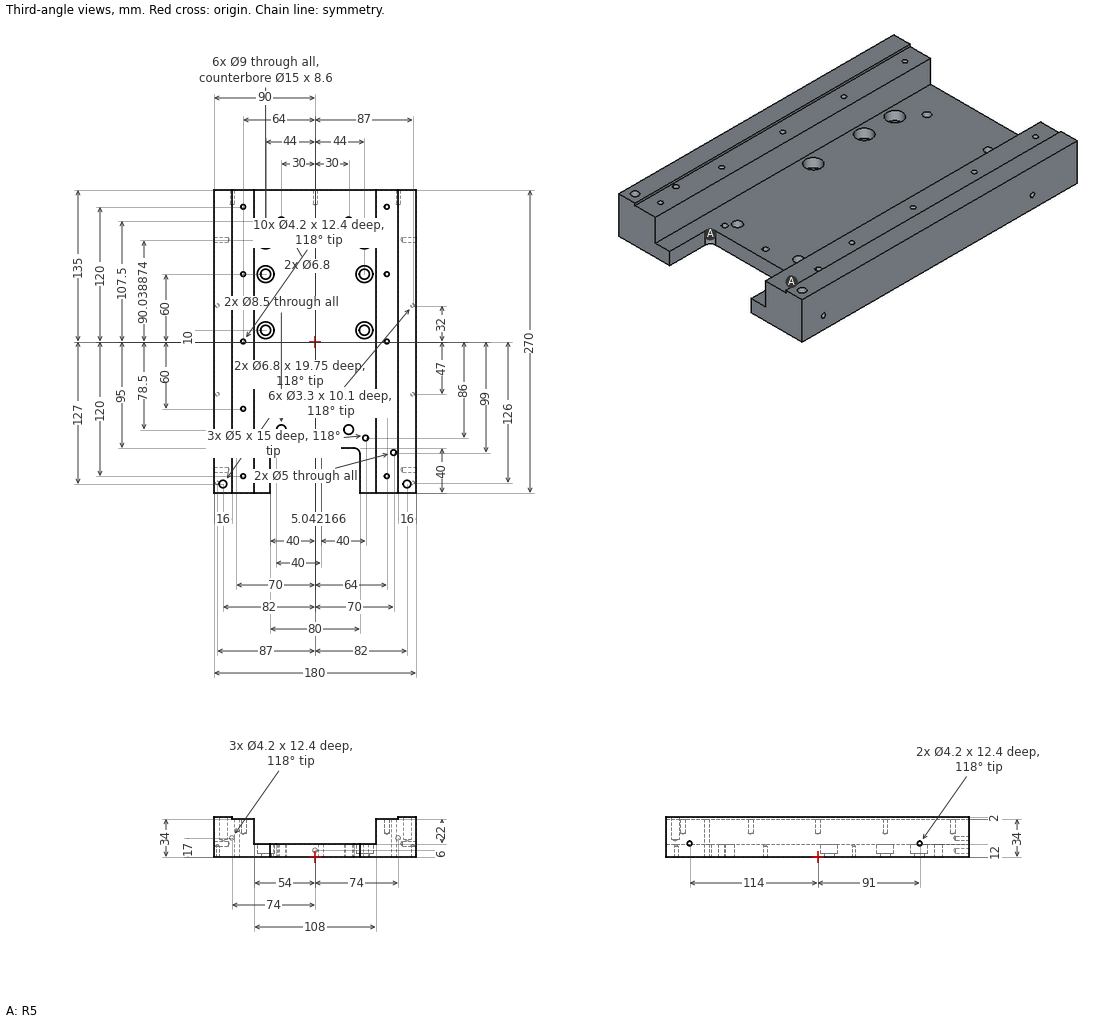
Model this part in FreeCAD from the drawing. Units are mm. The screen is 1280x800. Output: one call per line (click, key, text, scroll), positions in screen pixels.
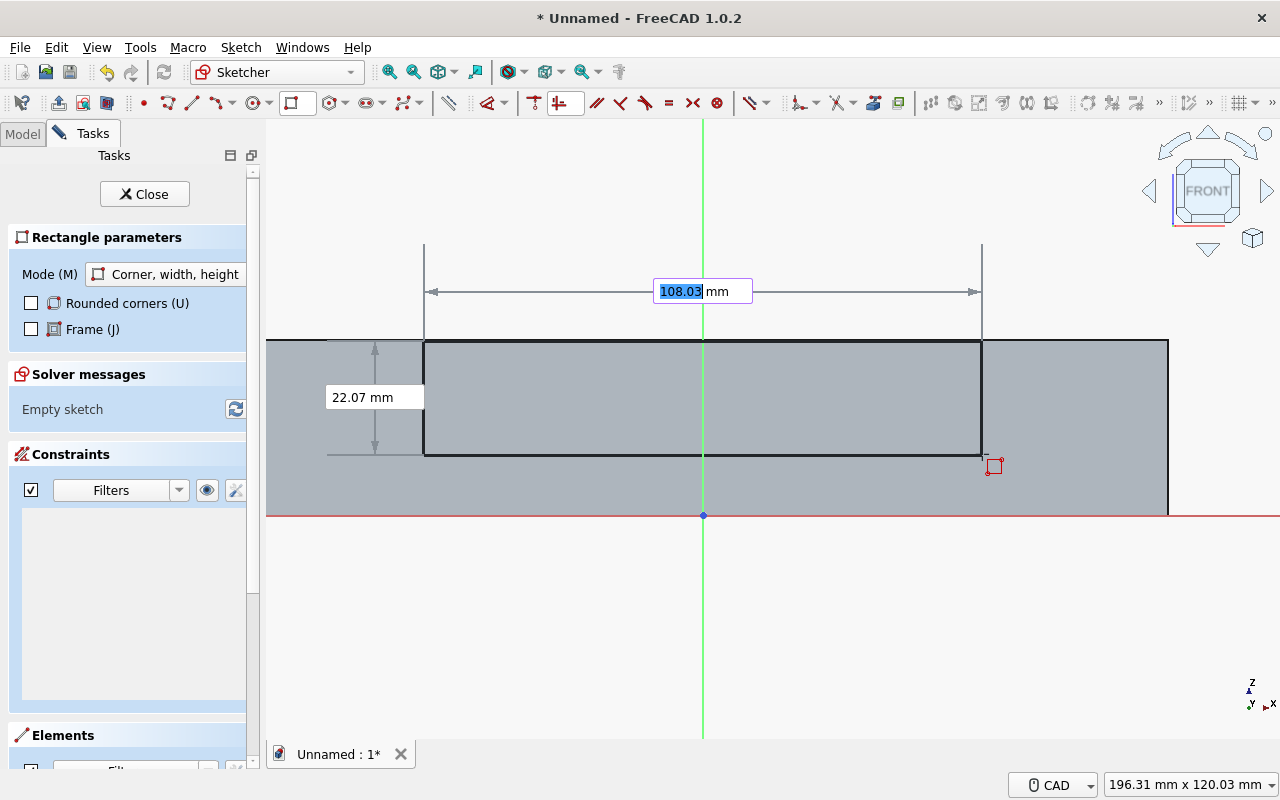
text(108)
key(Tab)
text(22)
key(Return)
key(Escape)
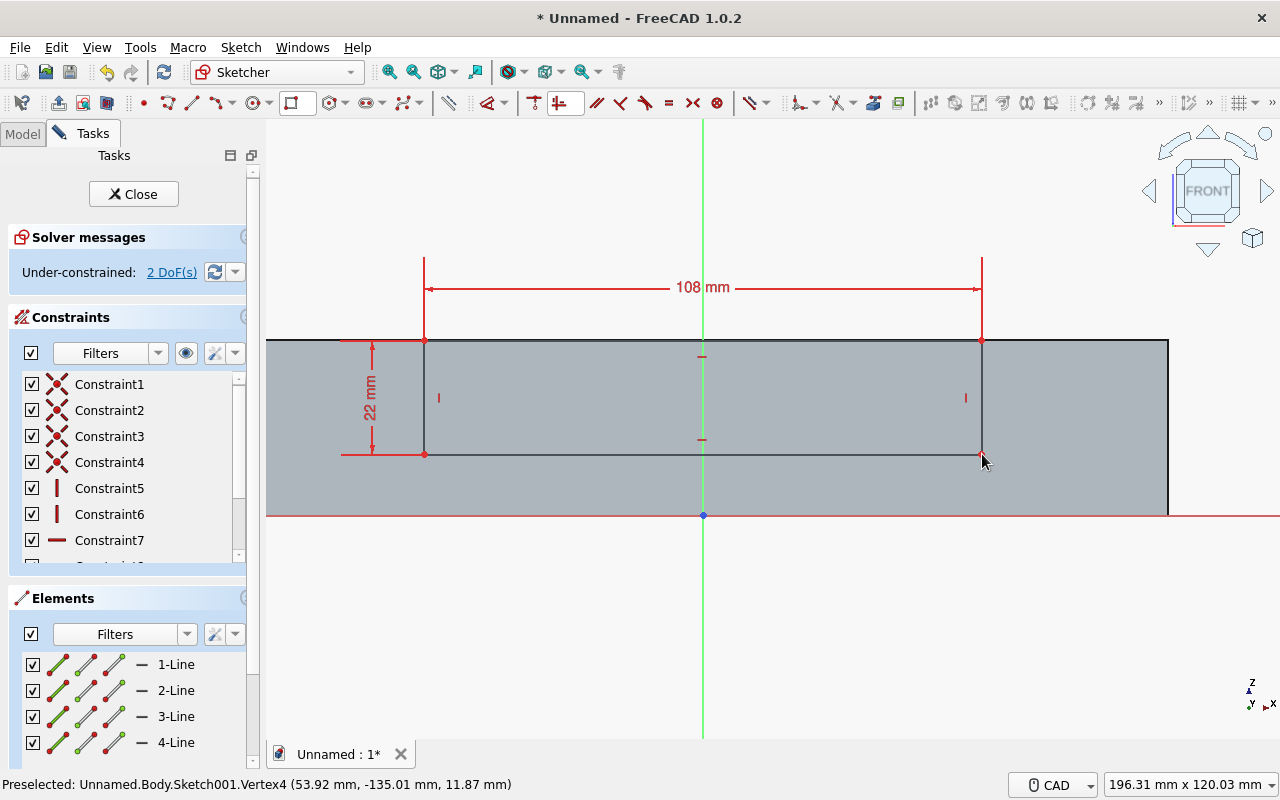
click(488, 104)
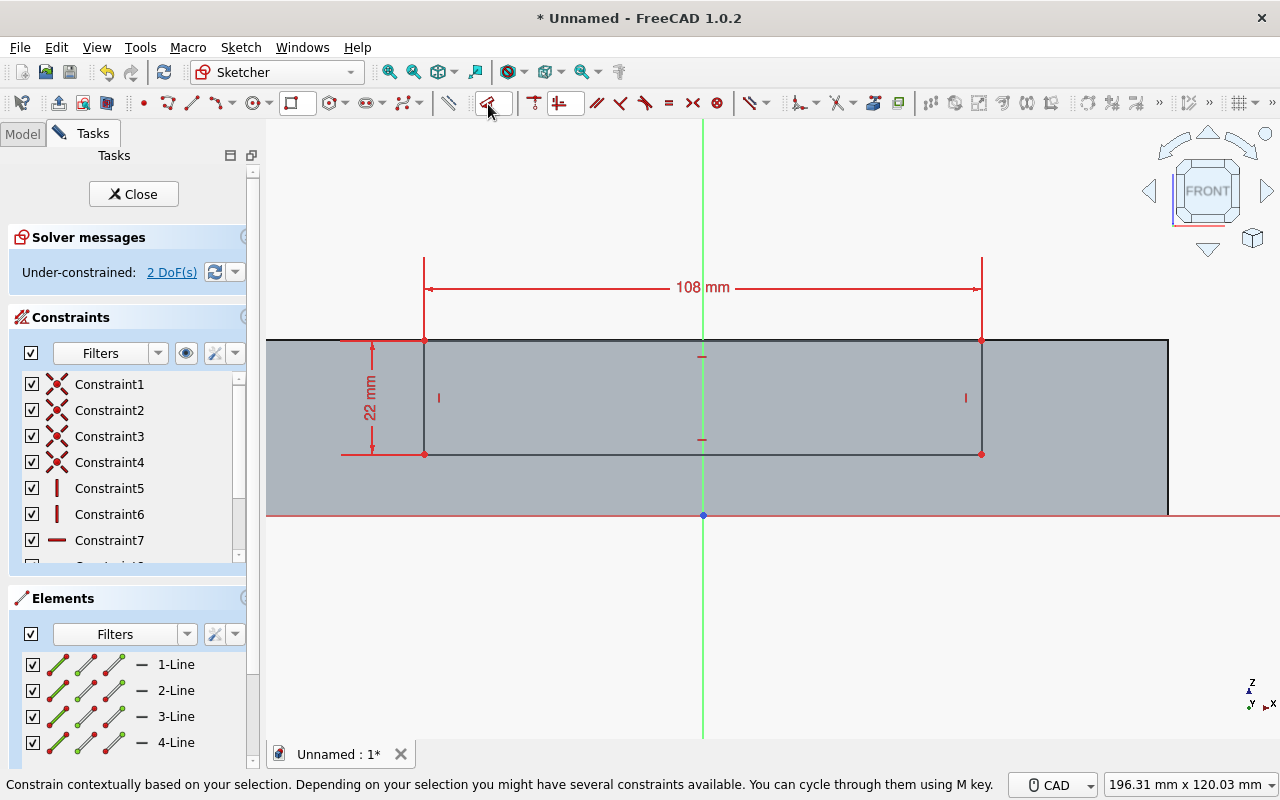
click(424, 341)
click(564, 550)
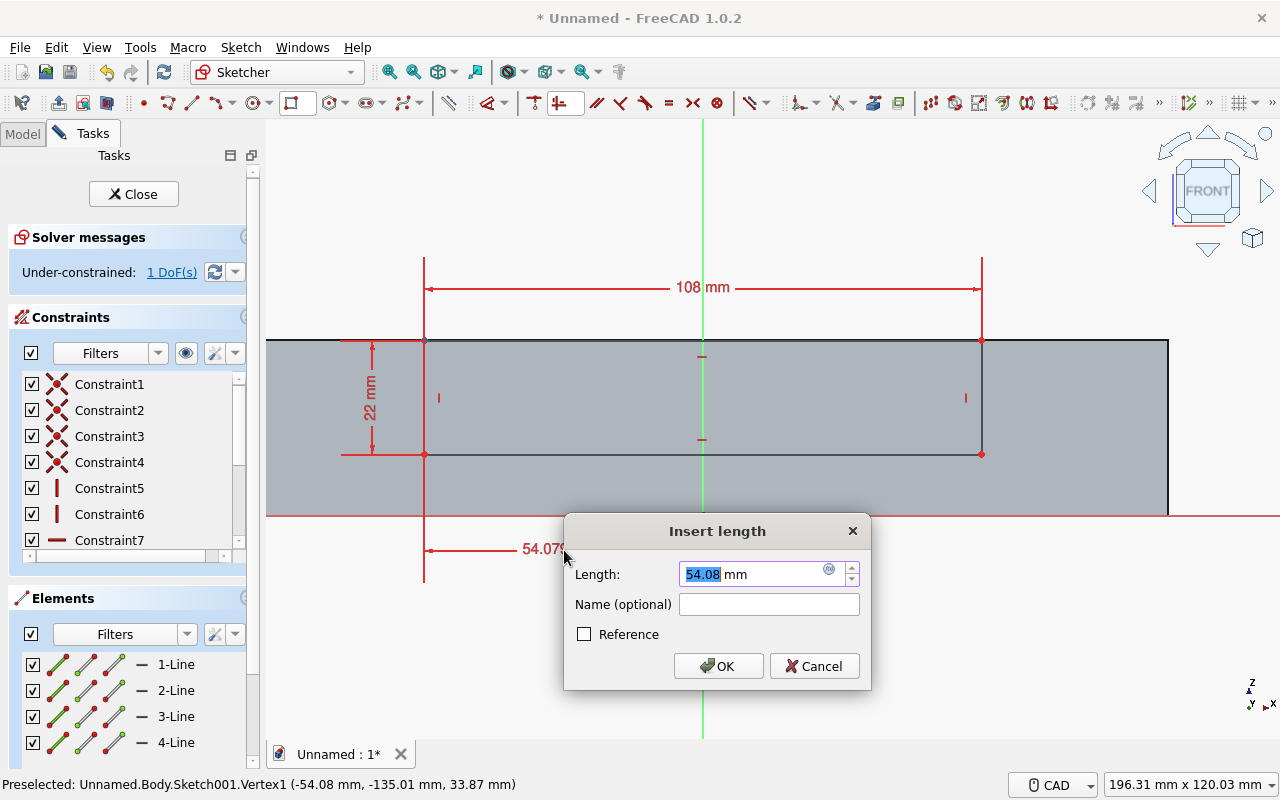
text(54)
key(Return)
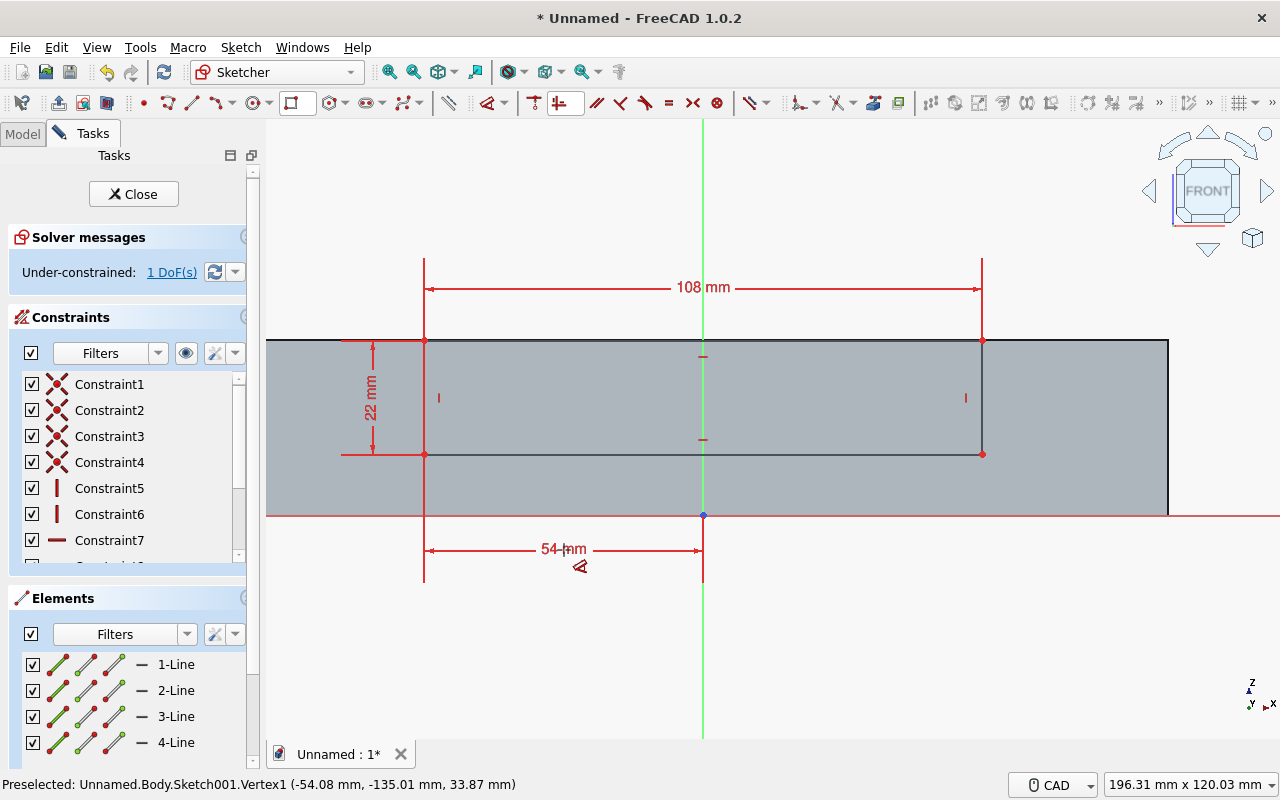
click(424, 341)
click(390, 428)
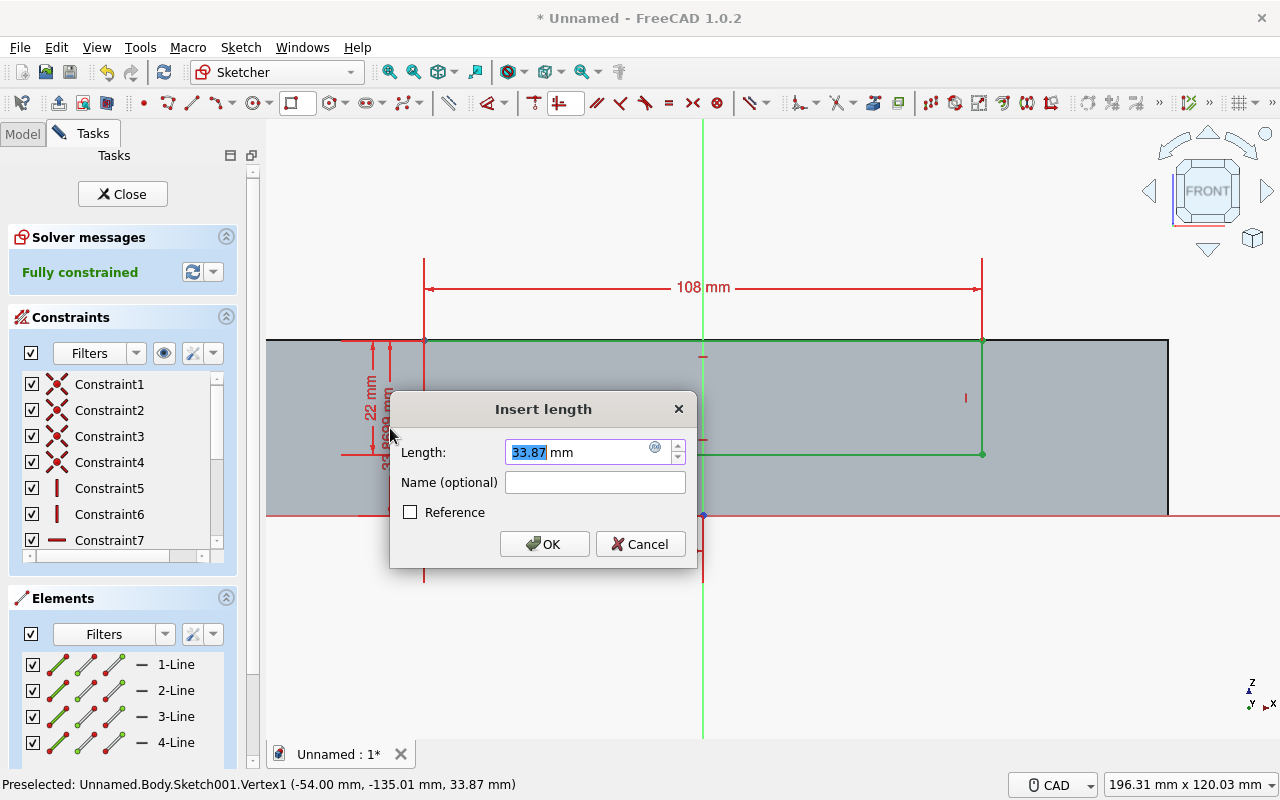
text(34)
key(Return)
key(Escape)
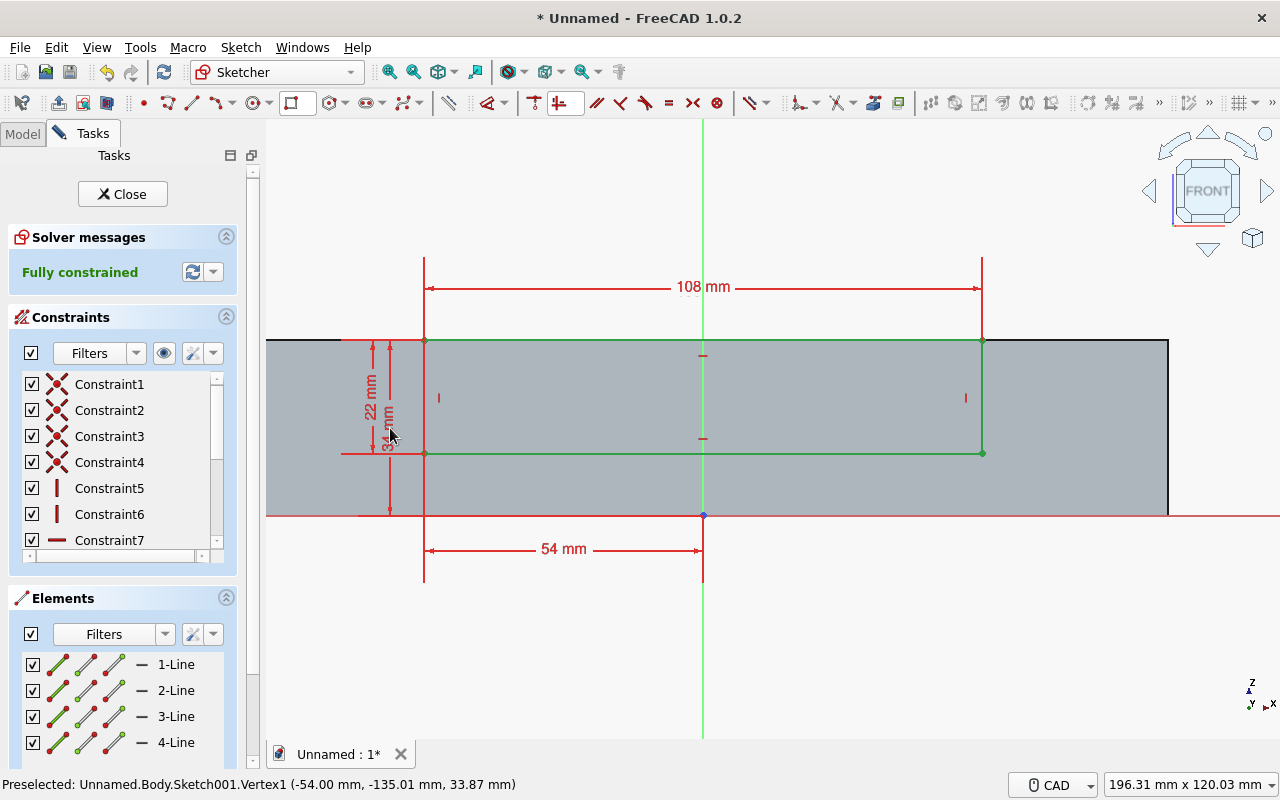
click(123, 194)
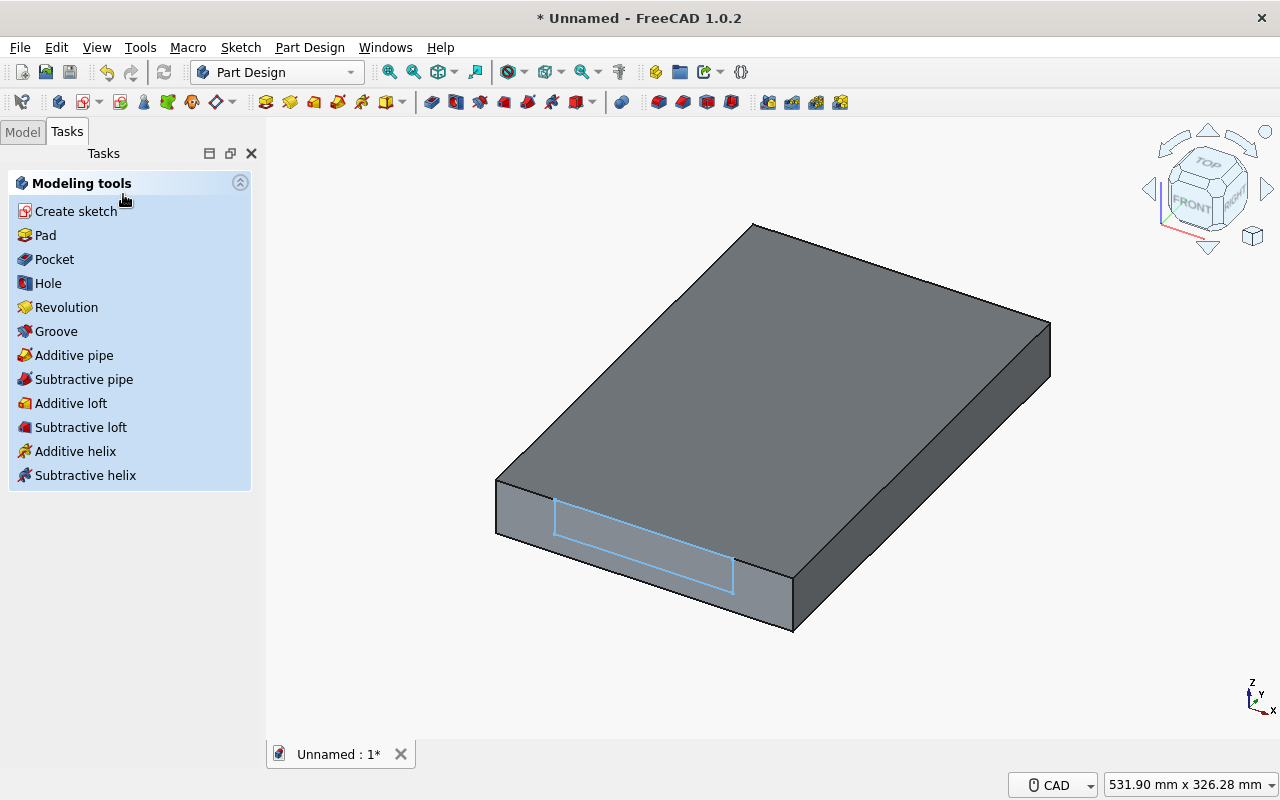
click(432, 102)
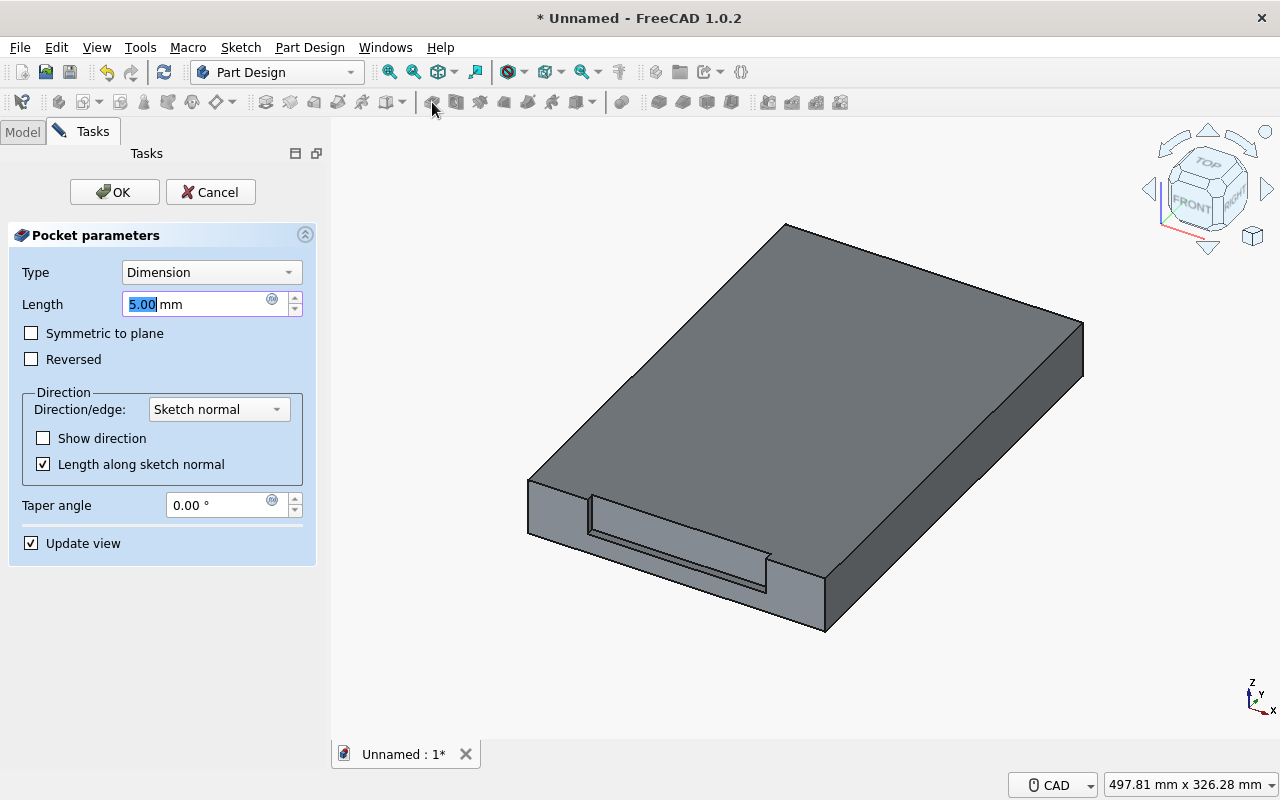
click(212, 272)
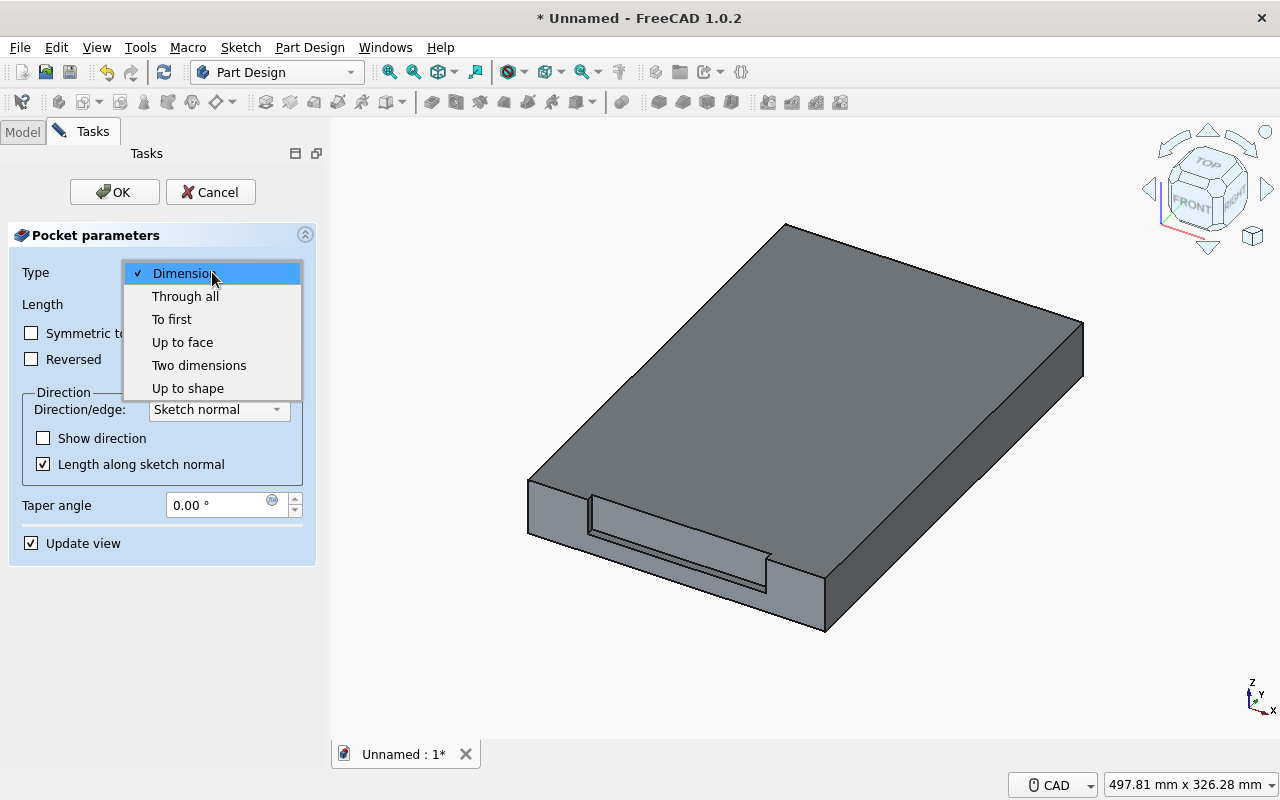
click(212, 296)